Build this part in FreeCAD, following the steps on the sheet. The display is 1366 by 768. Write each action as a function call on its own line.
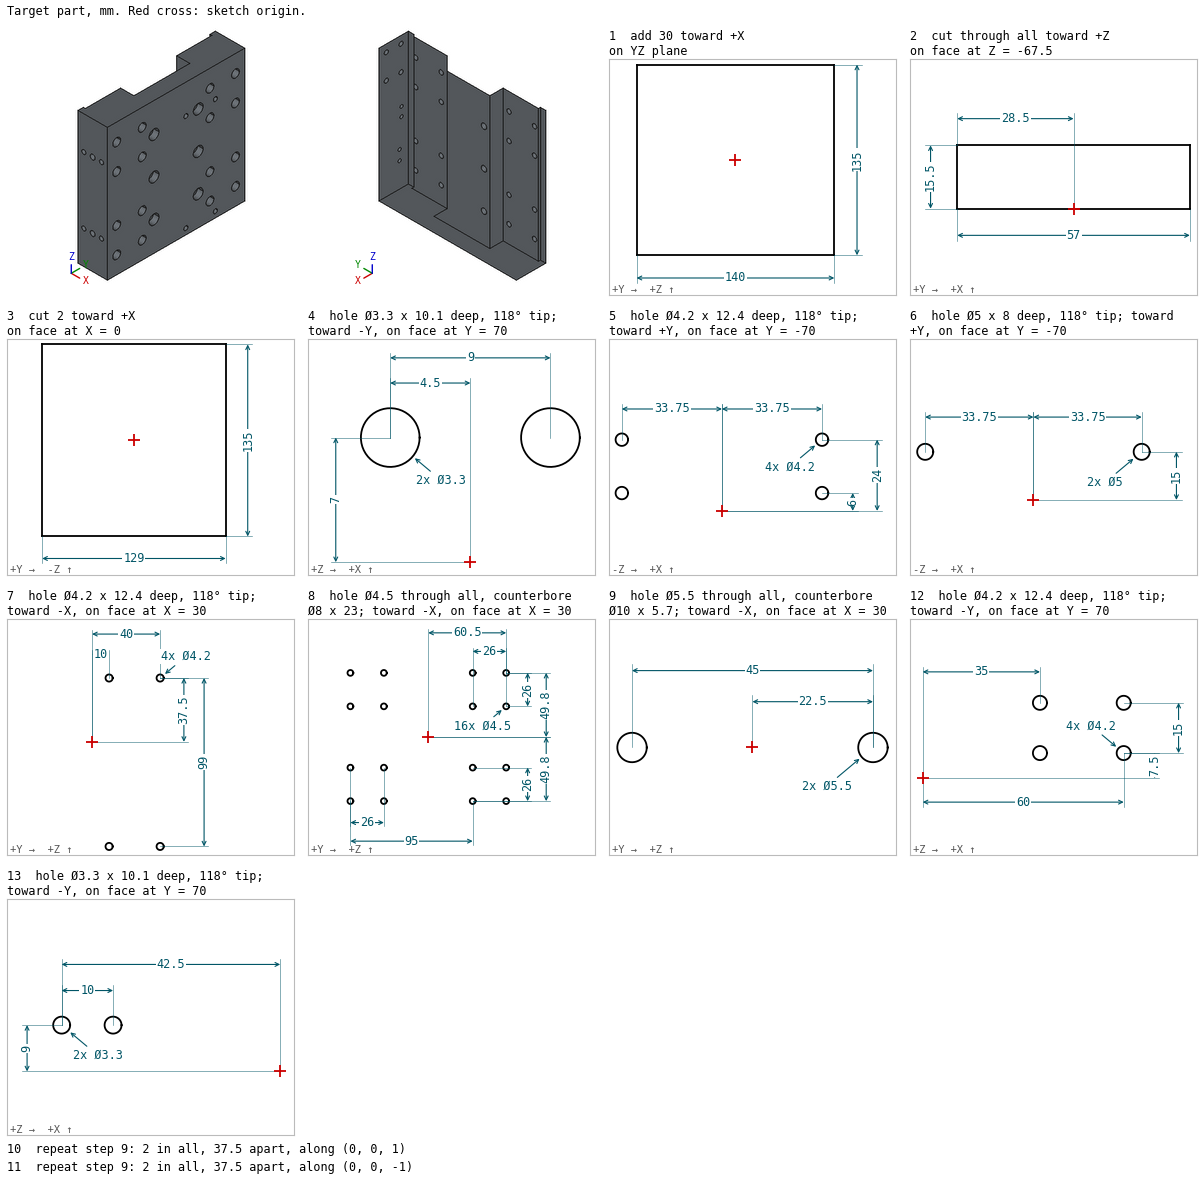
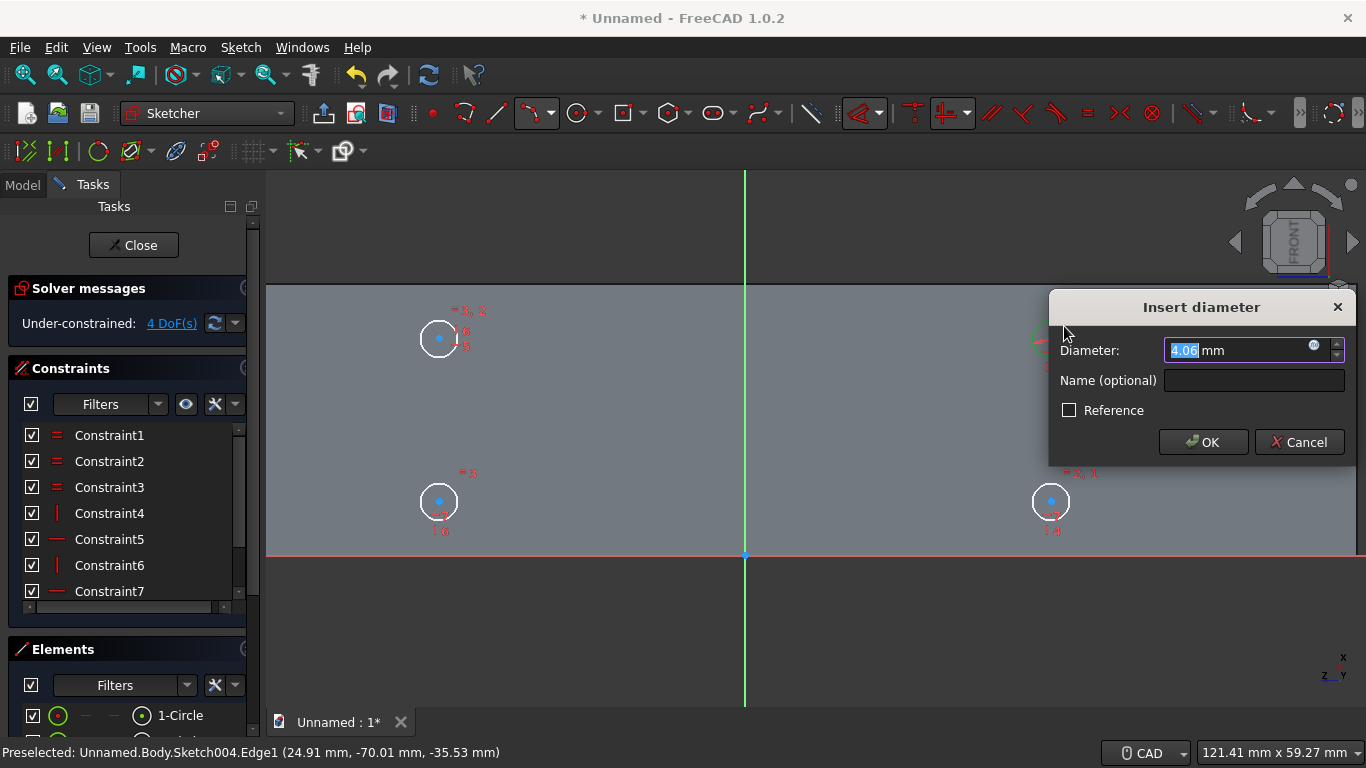
text(4.2)
key(Return)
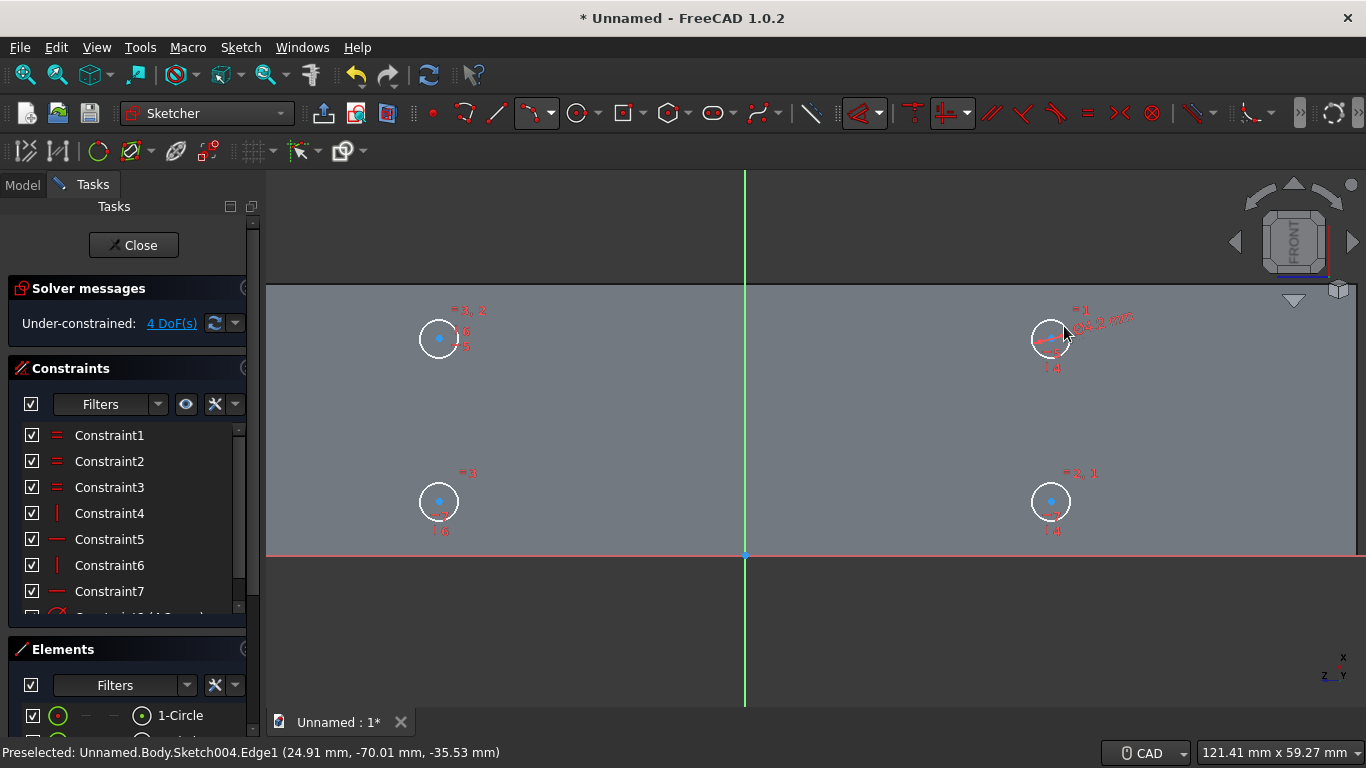
click(1051, 502)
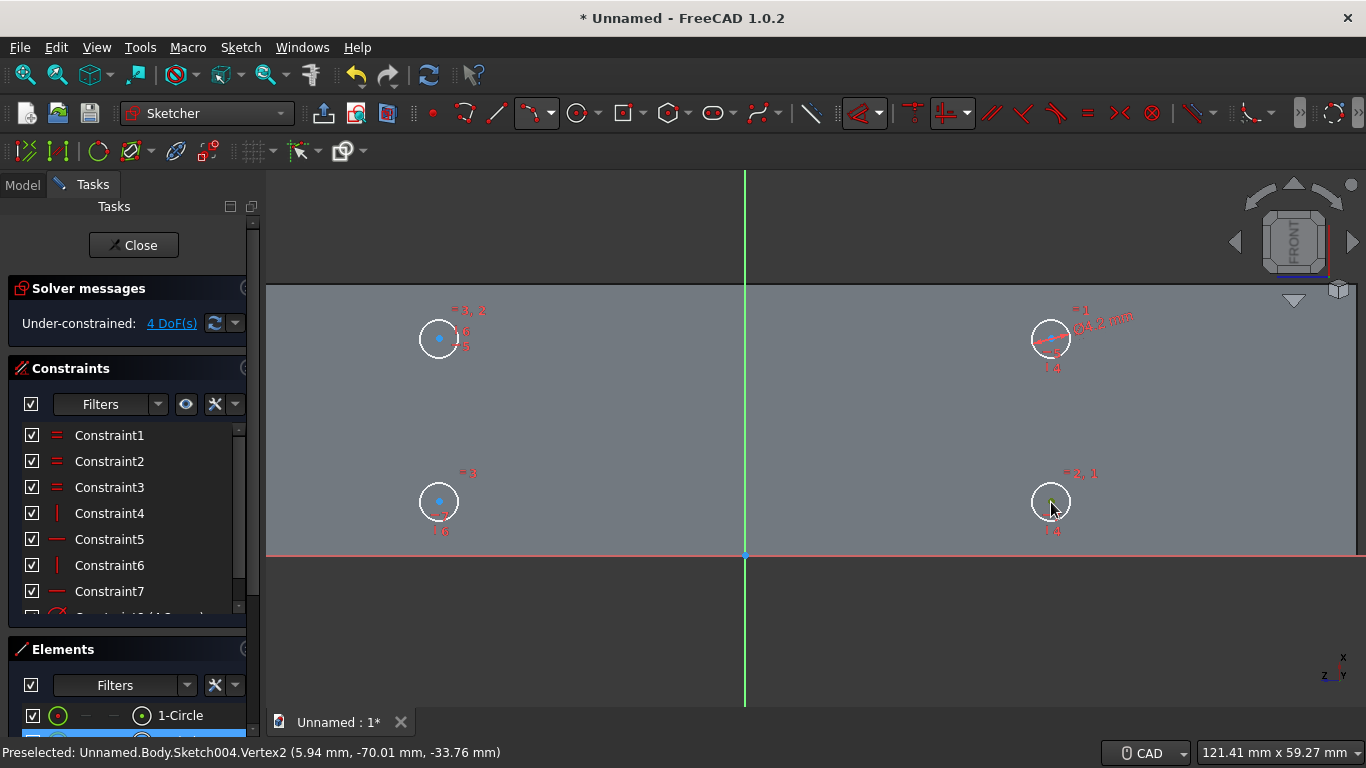
click(882, 114)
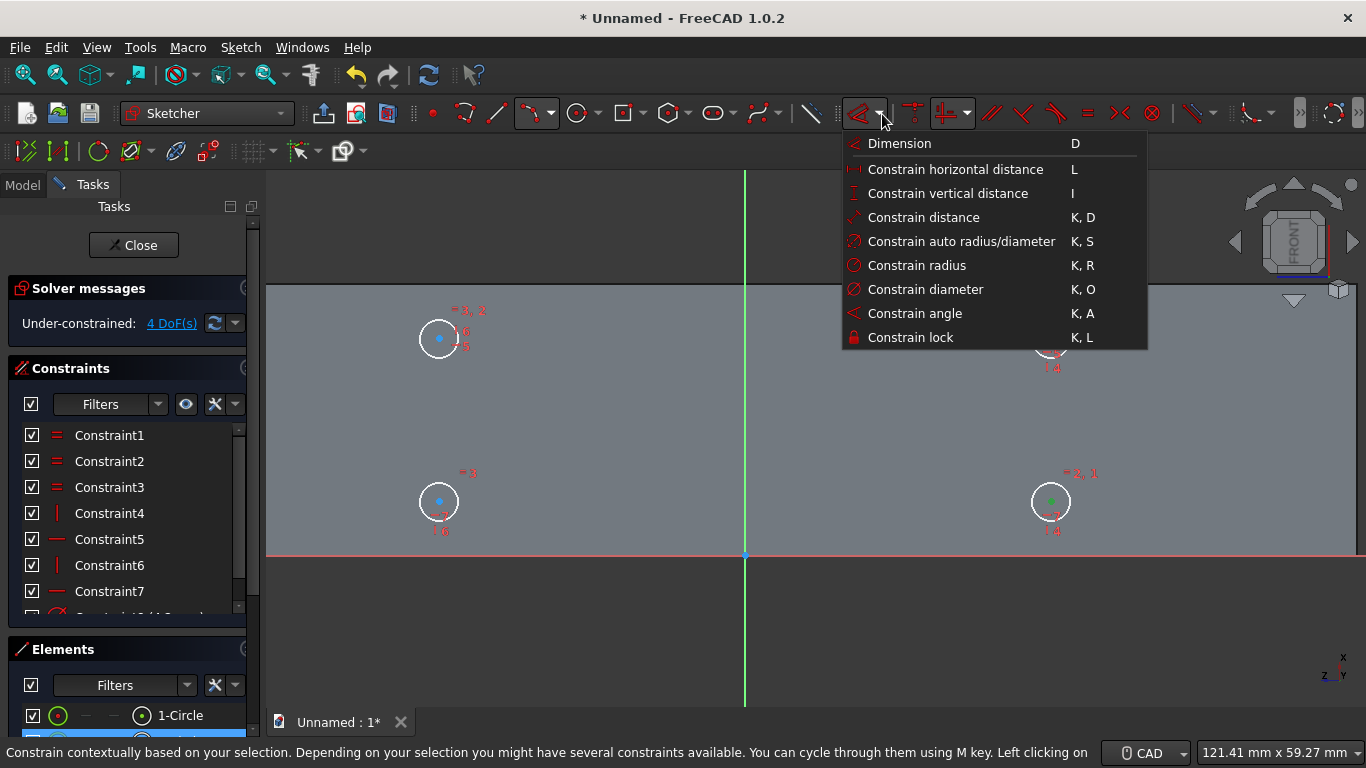
click(995, 193)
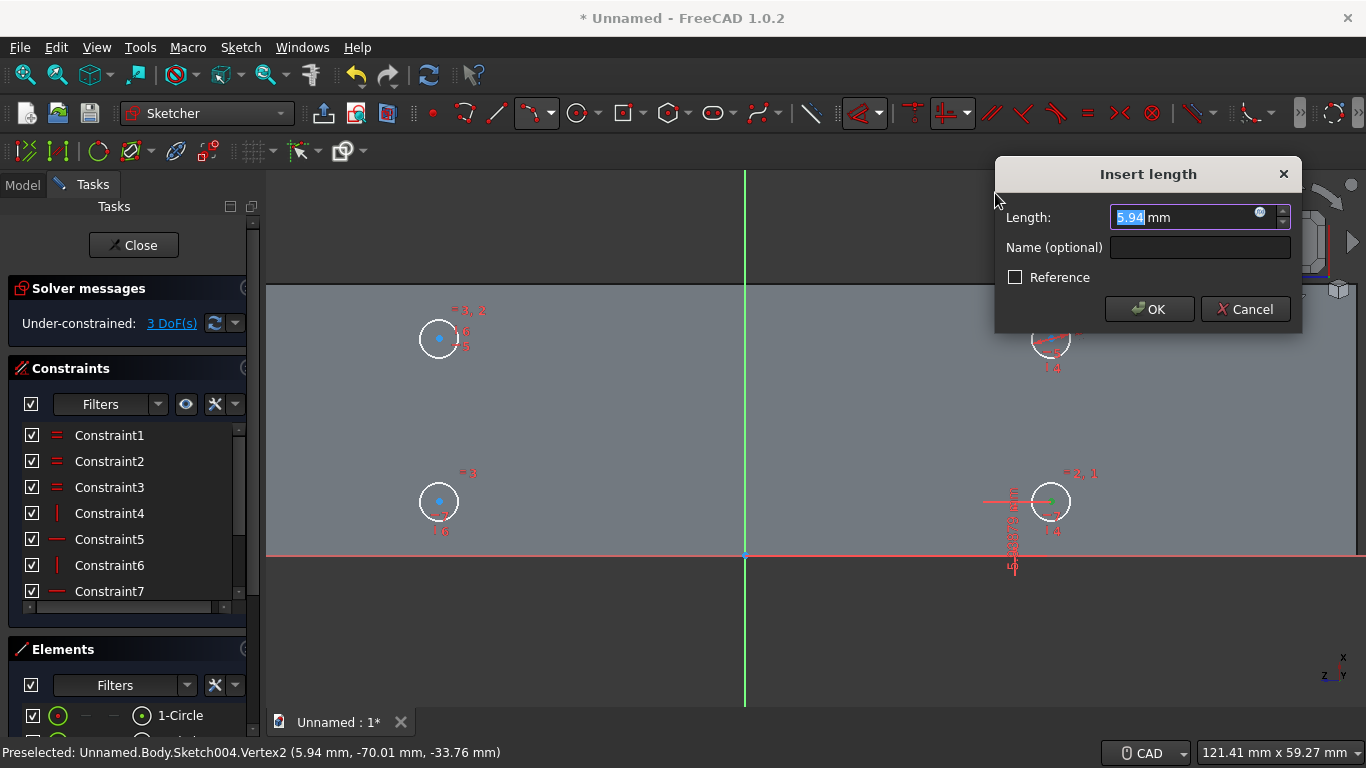
text(6)
key(Return)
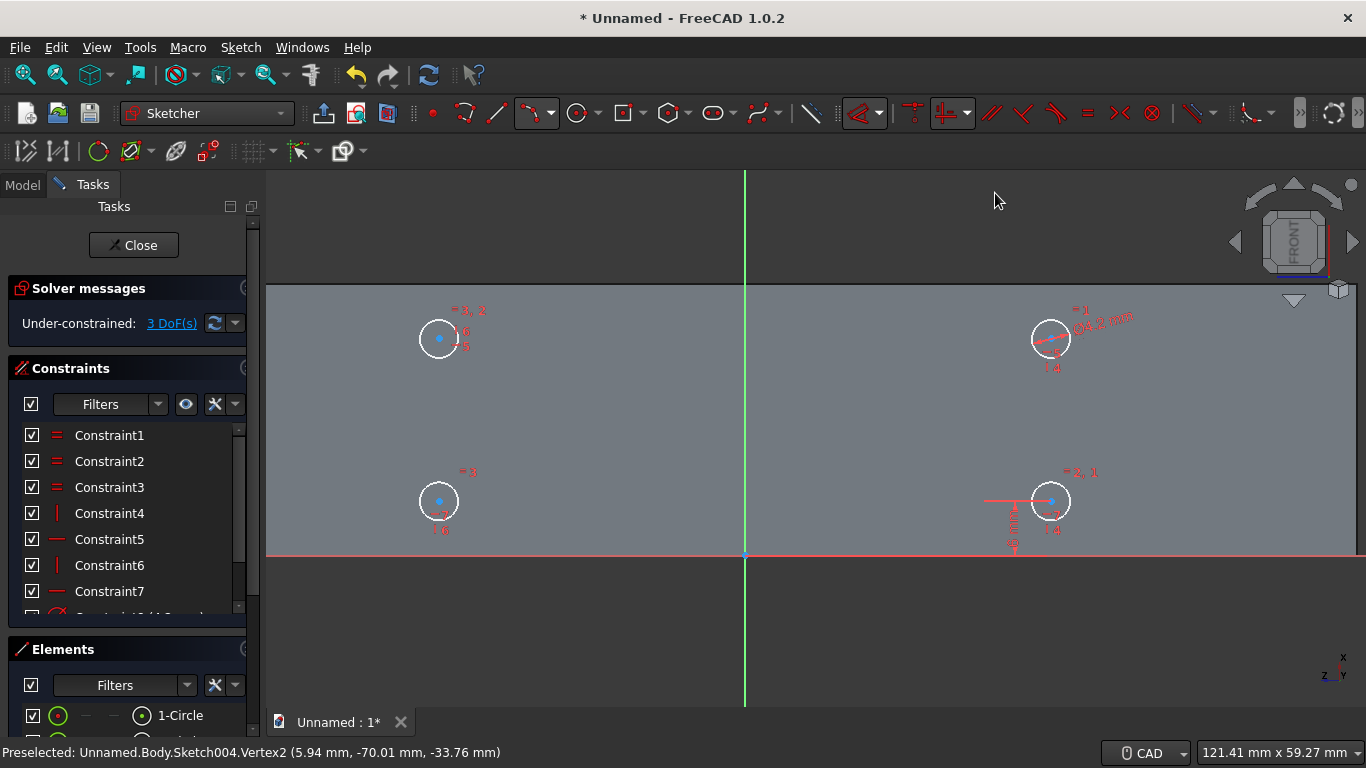
click(1051, 339)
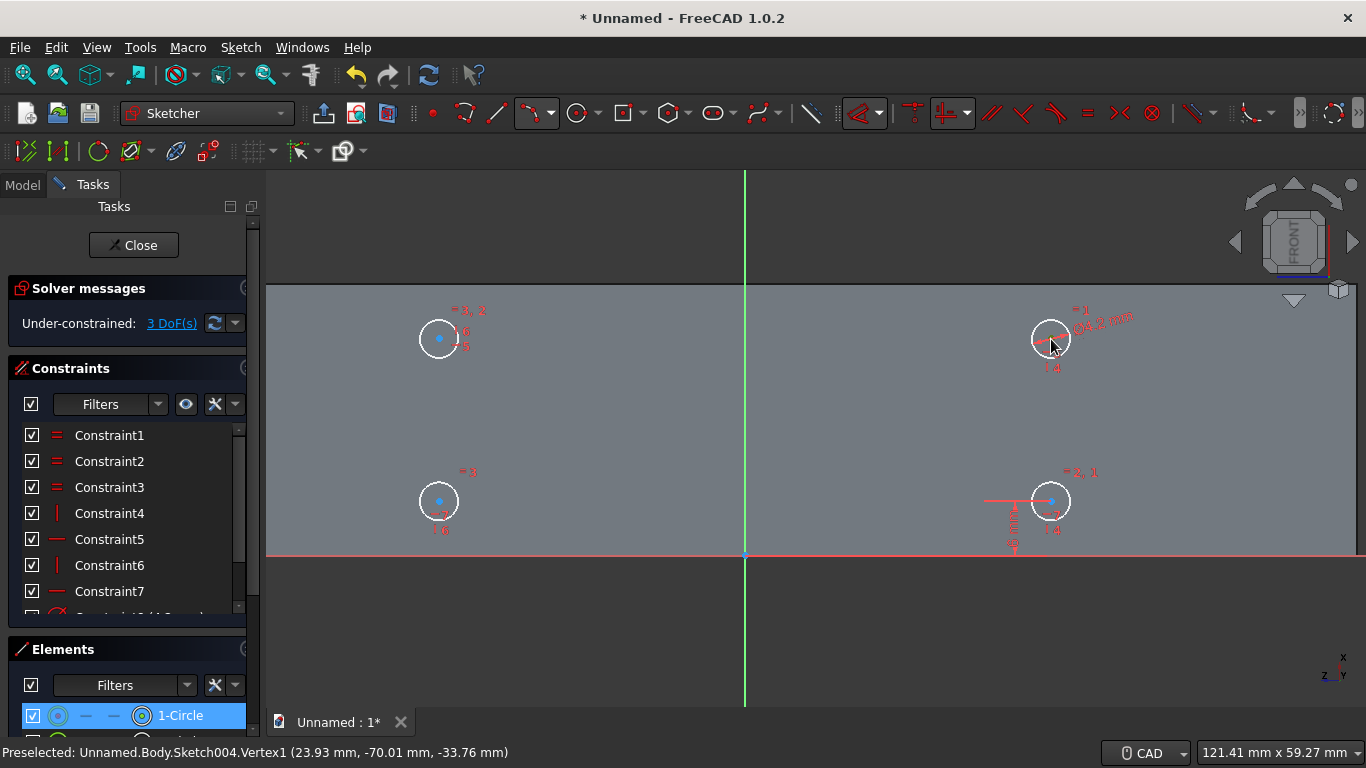
click(882, 114)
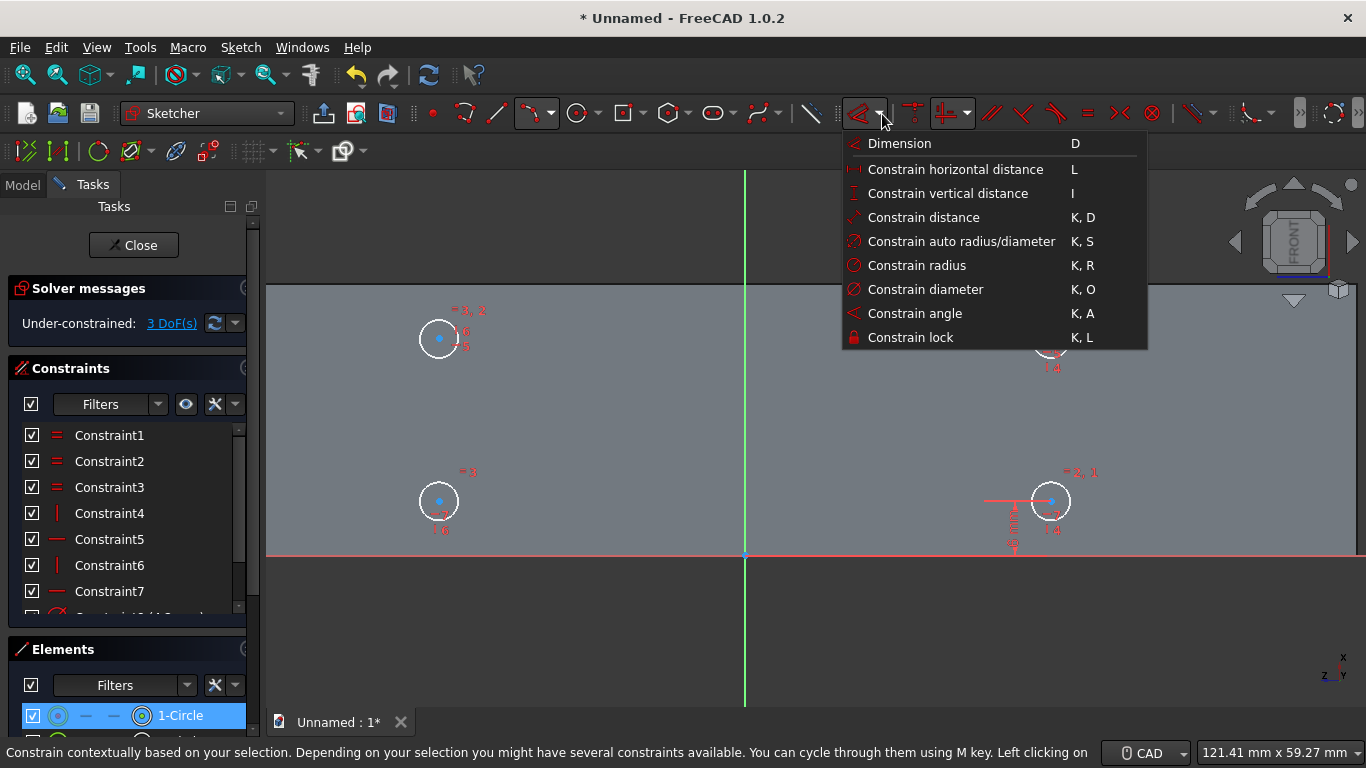
click(995, 193)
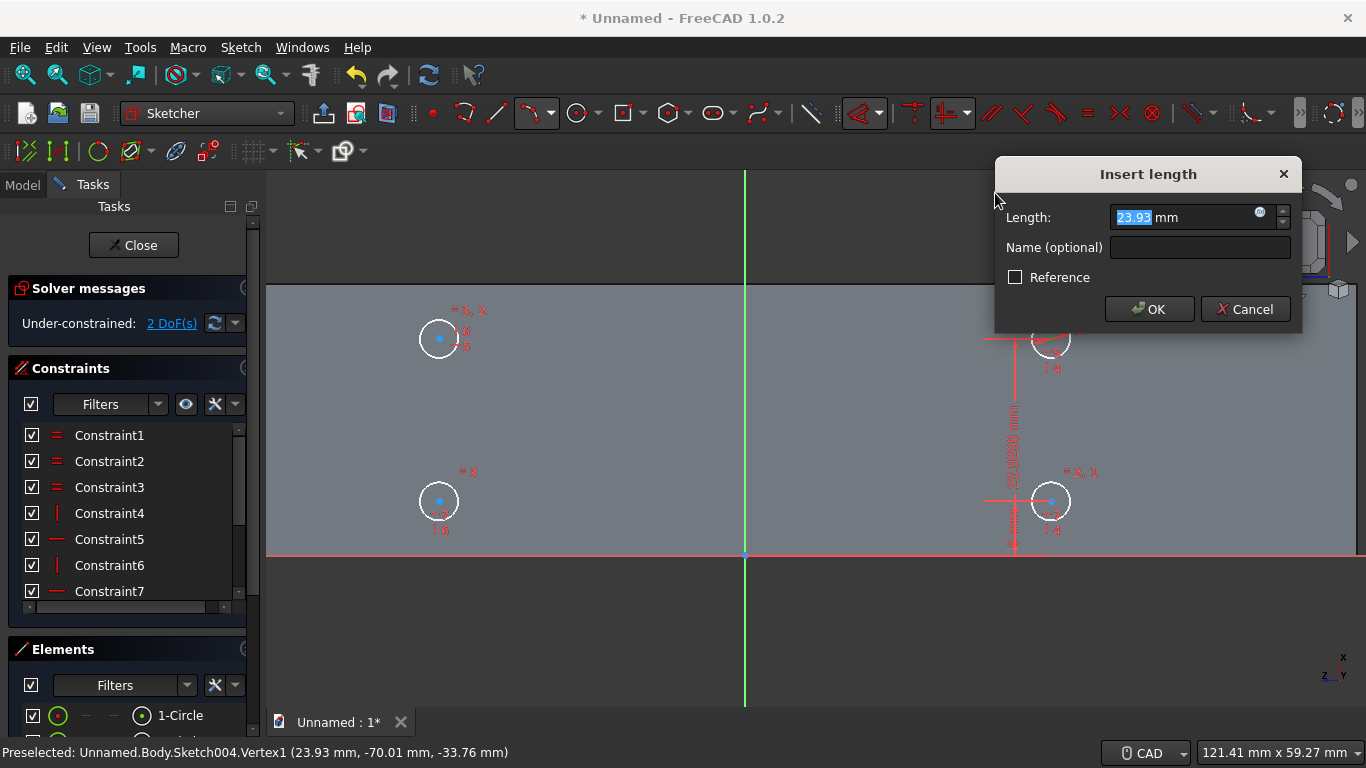
text(24)
key(Return)